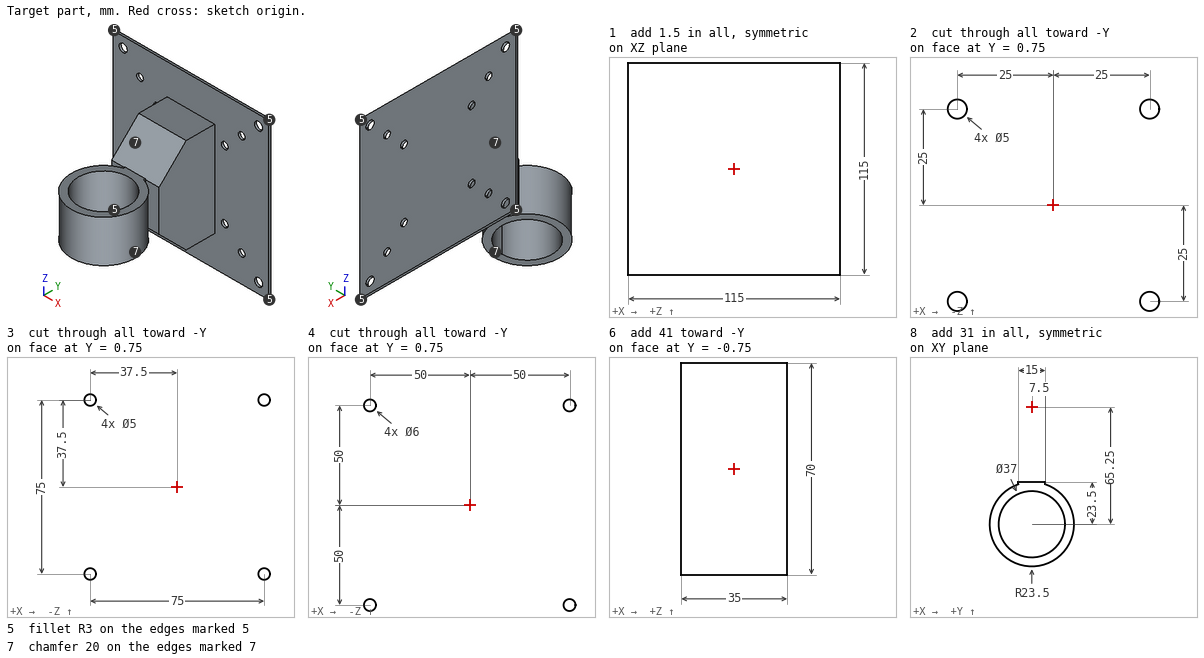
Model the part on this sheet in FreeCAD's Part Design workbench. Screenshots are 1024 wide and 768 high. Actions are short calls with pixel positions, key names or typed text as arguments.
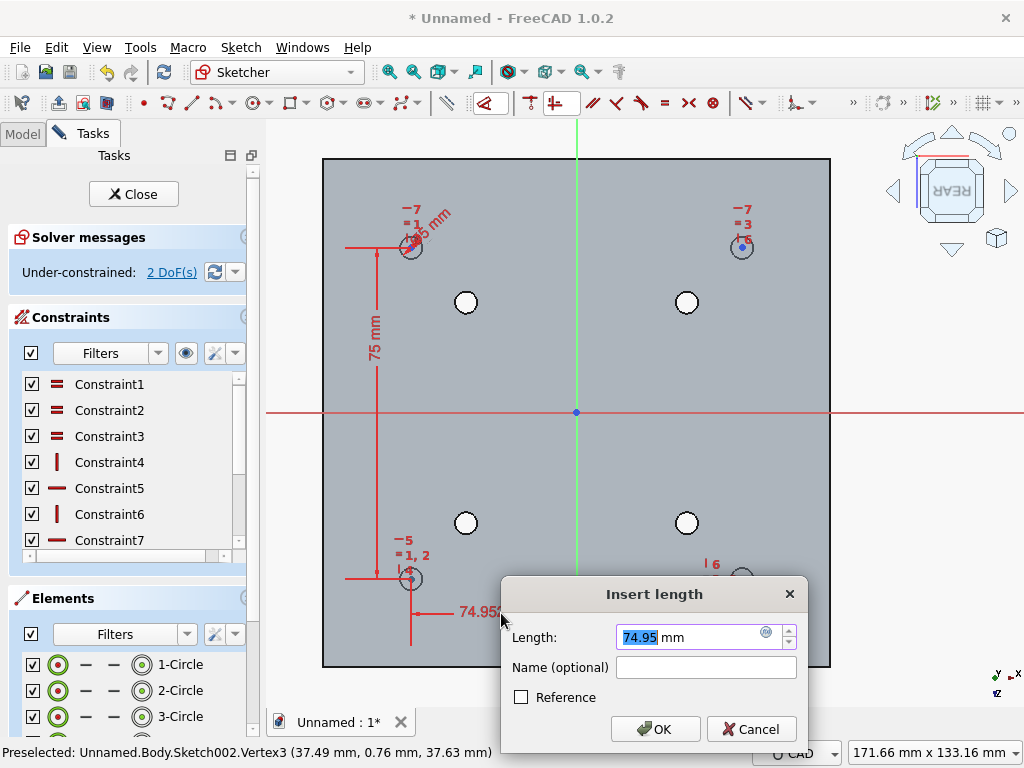
text(75)
key(Return)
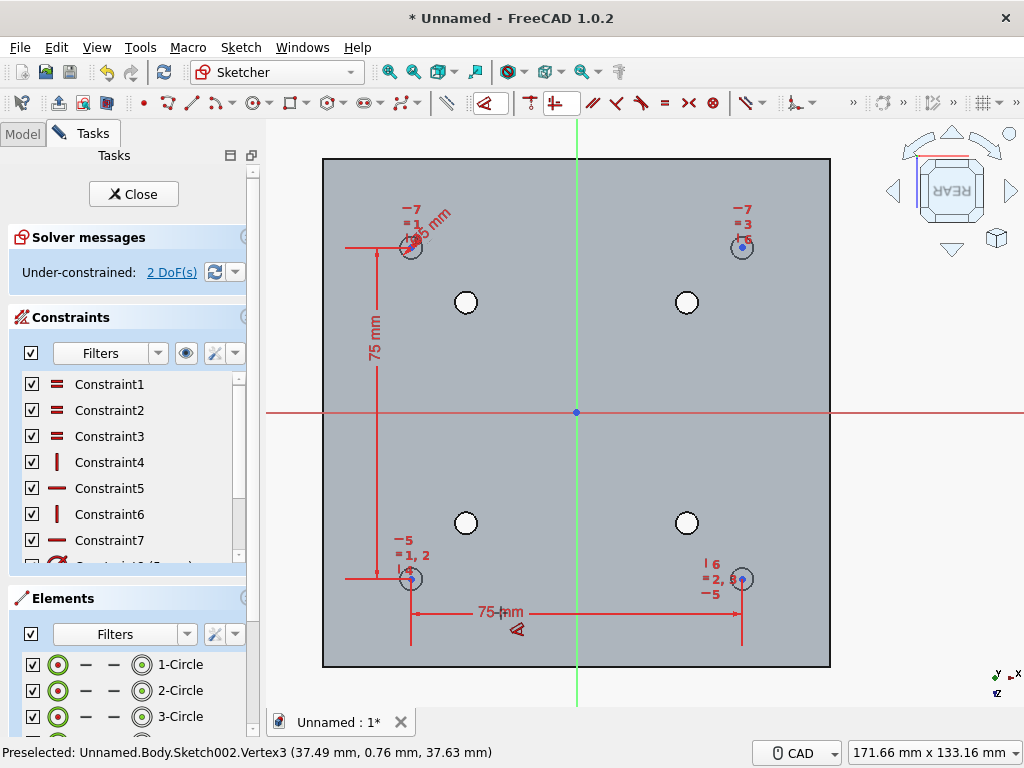
click(411, 248)
click(532, 214)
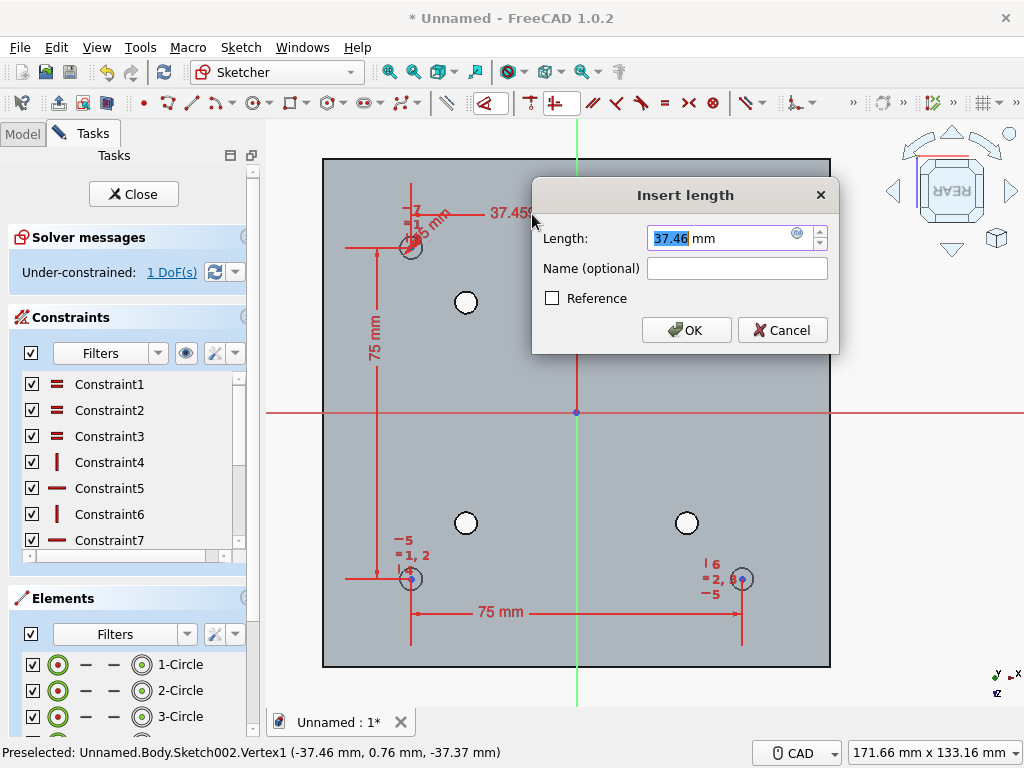
text(37.5)
key(Return)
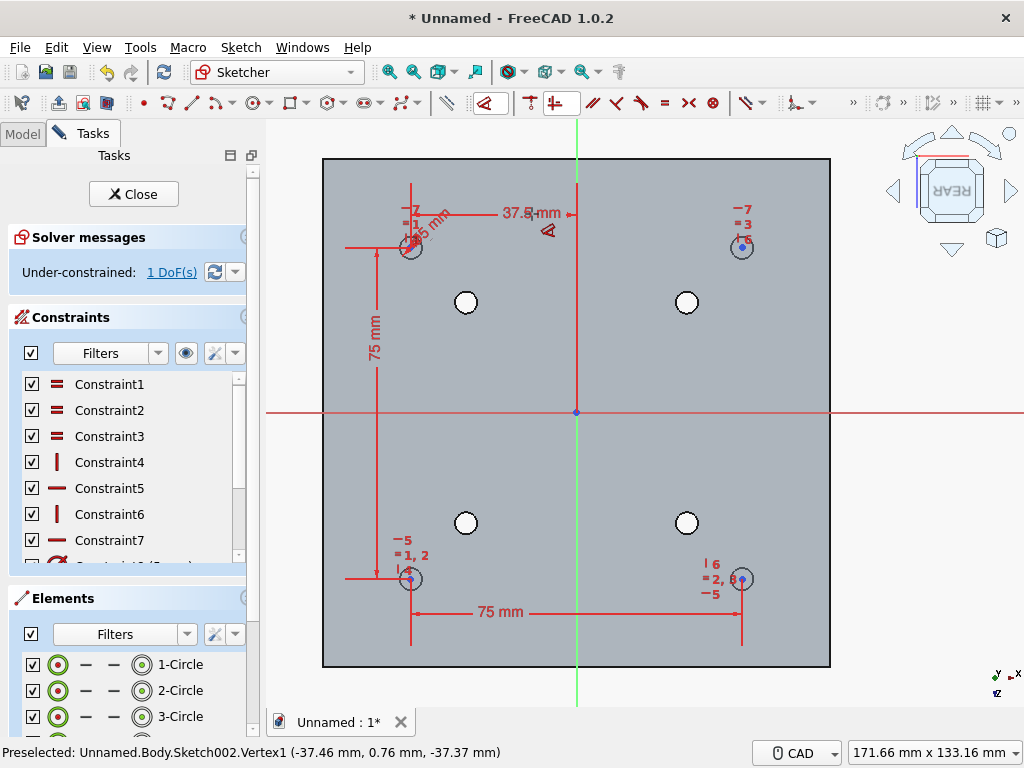
click(411, 248)
click(377, 292)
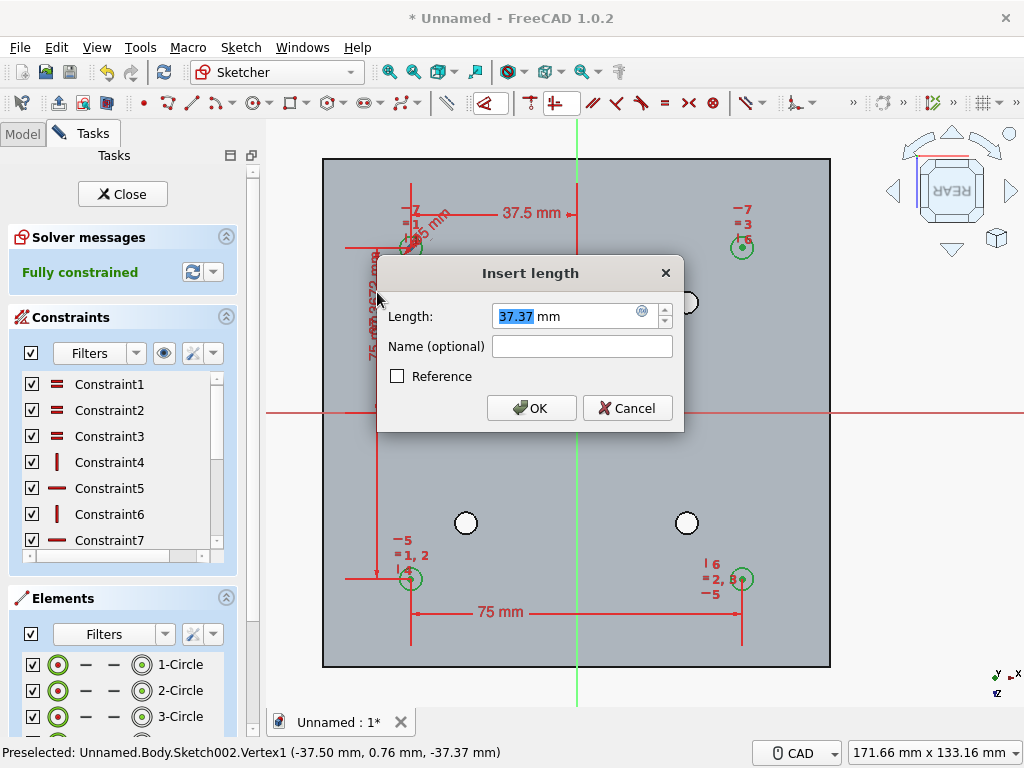
text(37.5)
key(Return)
key(Escape)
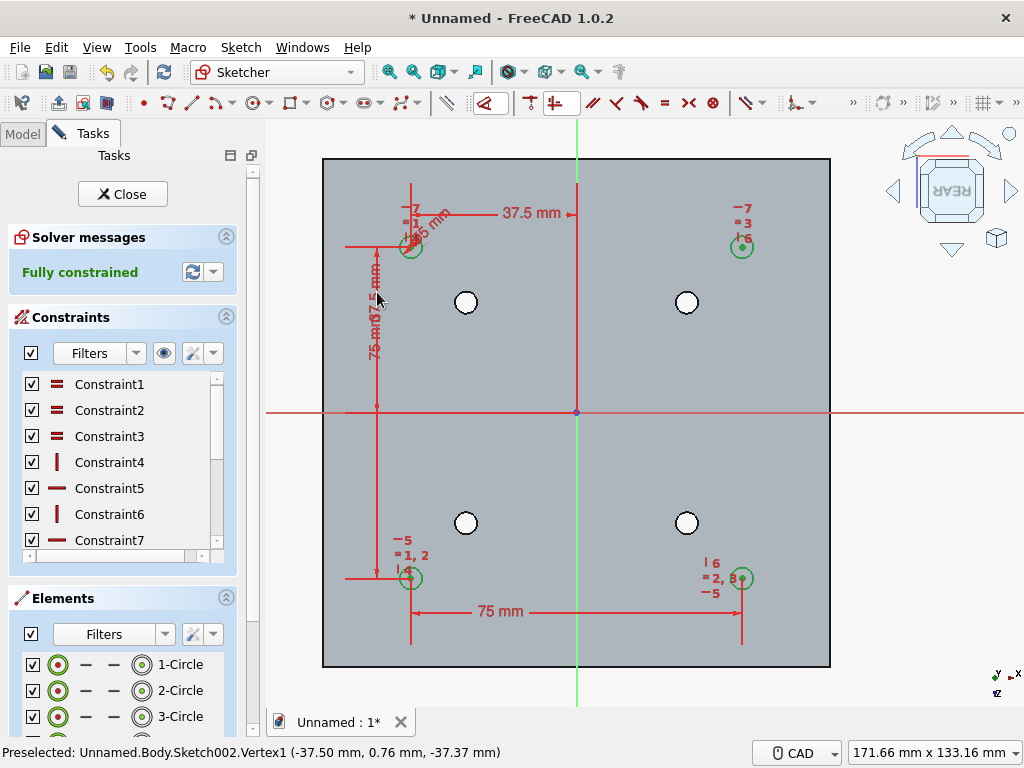
click(123, 194)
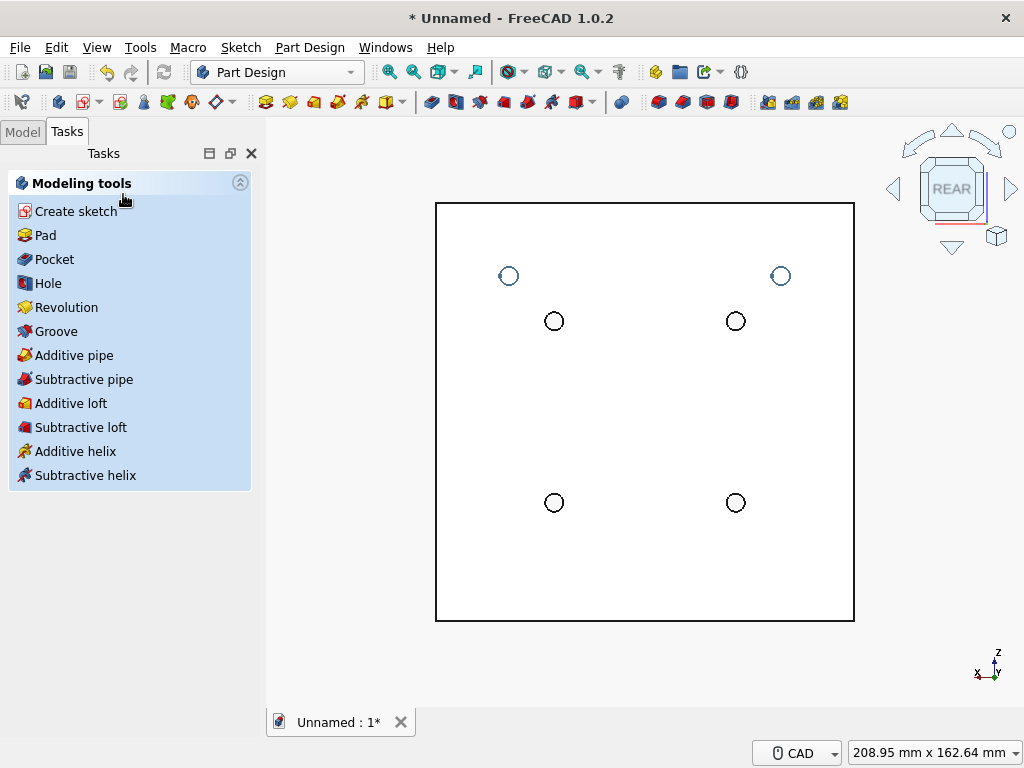
click(432, 102)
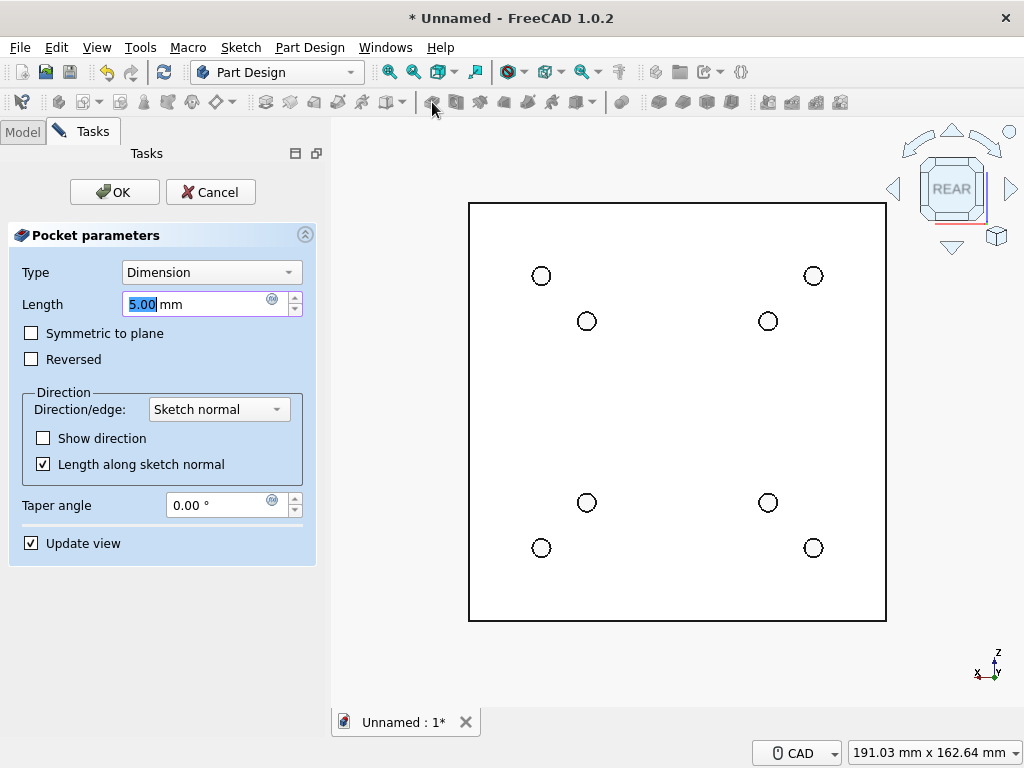
click(212, 272)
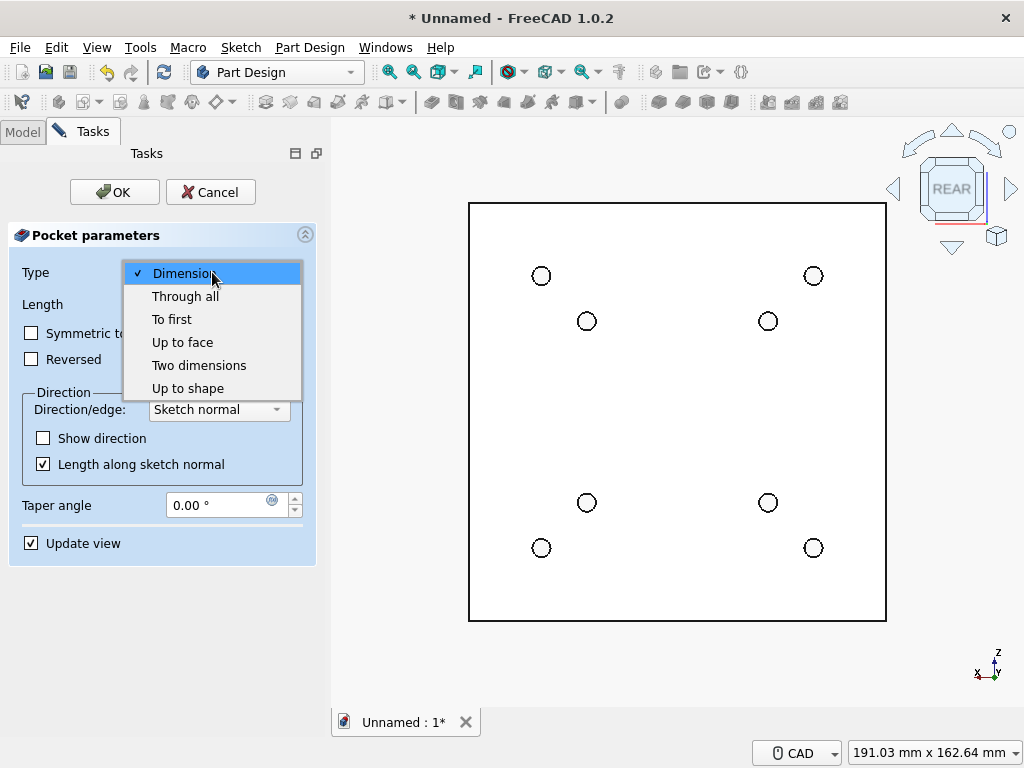
click(212, 296)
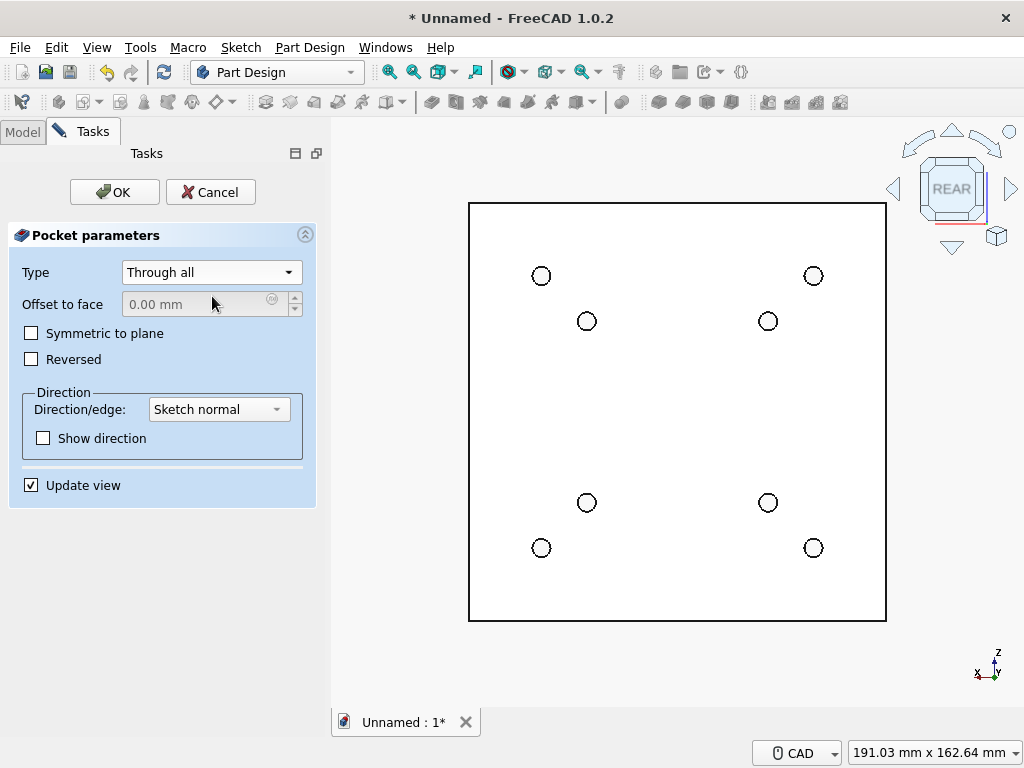
click(115, 192)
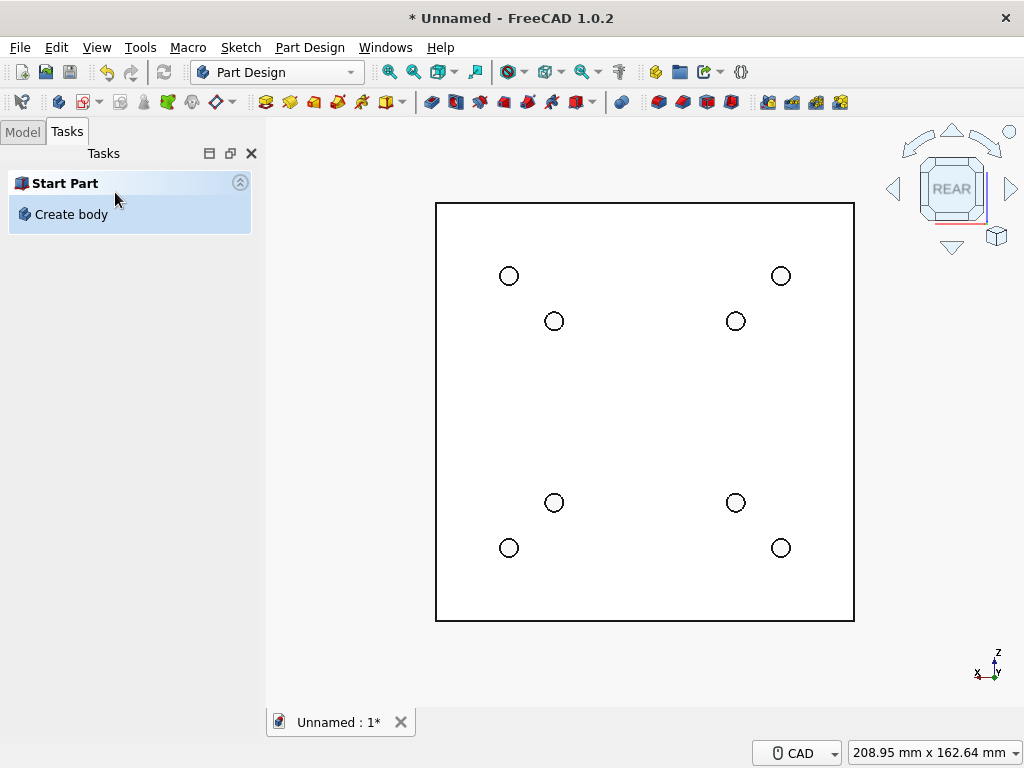
click(645, 411)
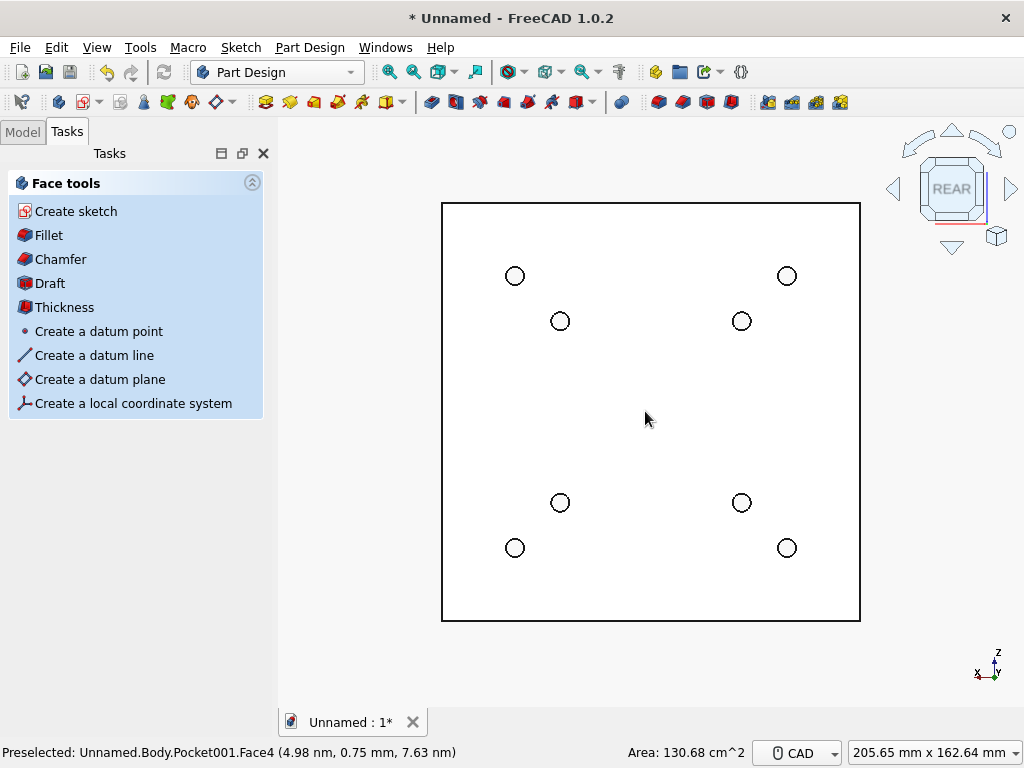
click(84, 102)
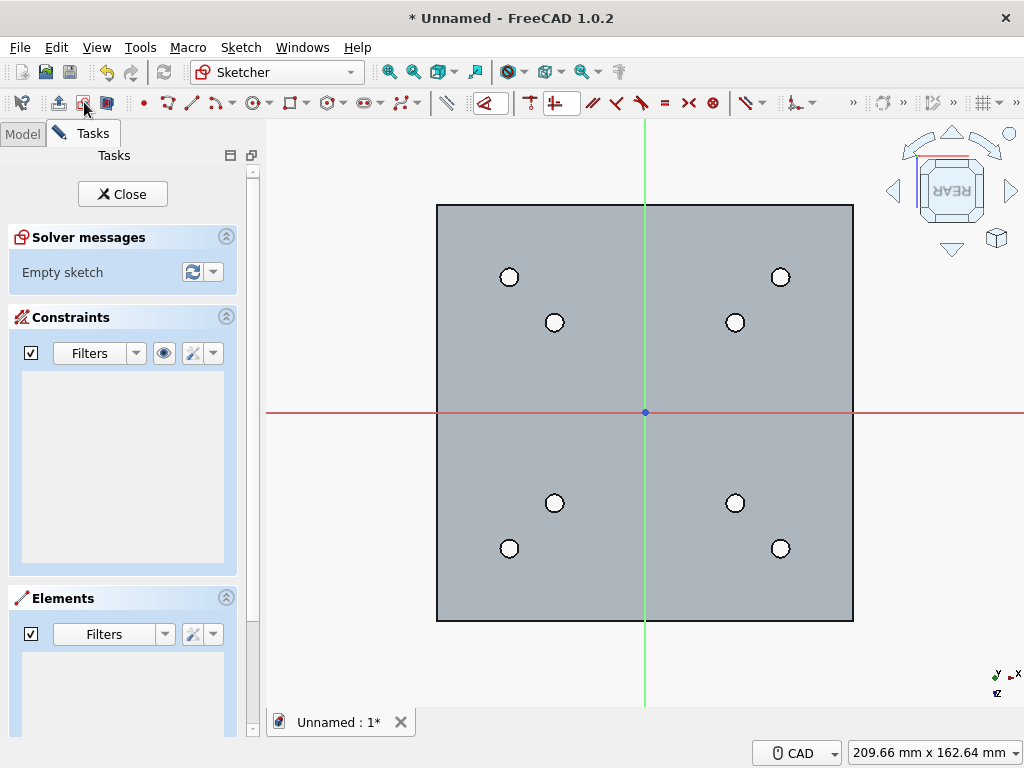
scroll(294, 413, down, 1)